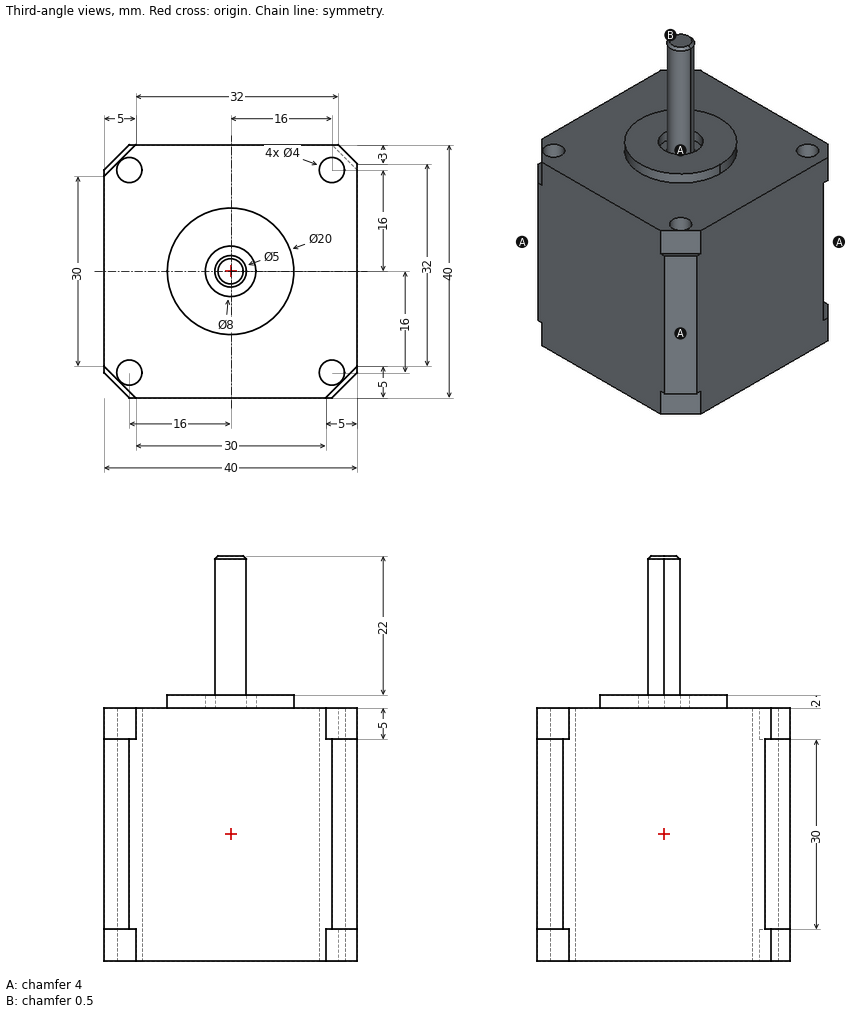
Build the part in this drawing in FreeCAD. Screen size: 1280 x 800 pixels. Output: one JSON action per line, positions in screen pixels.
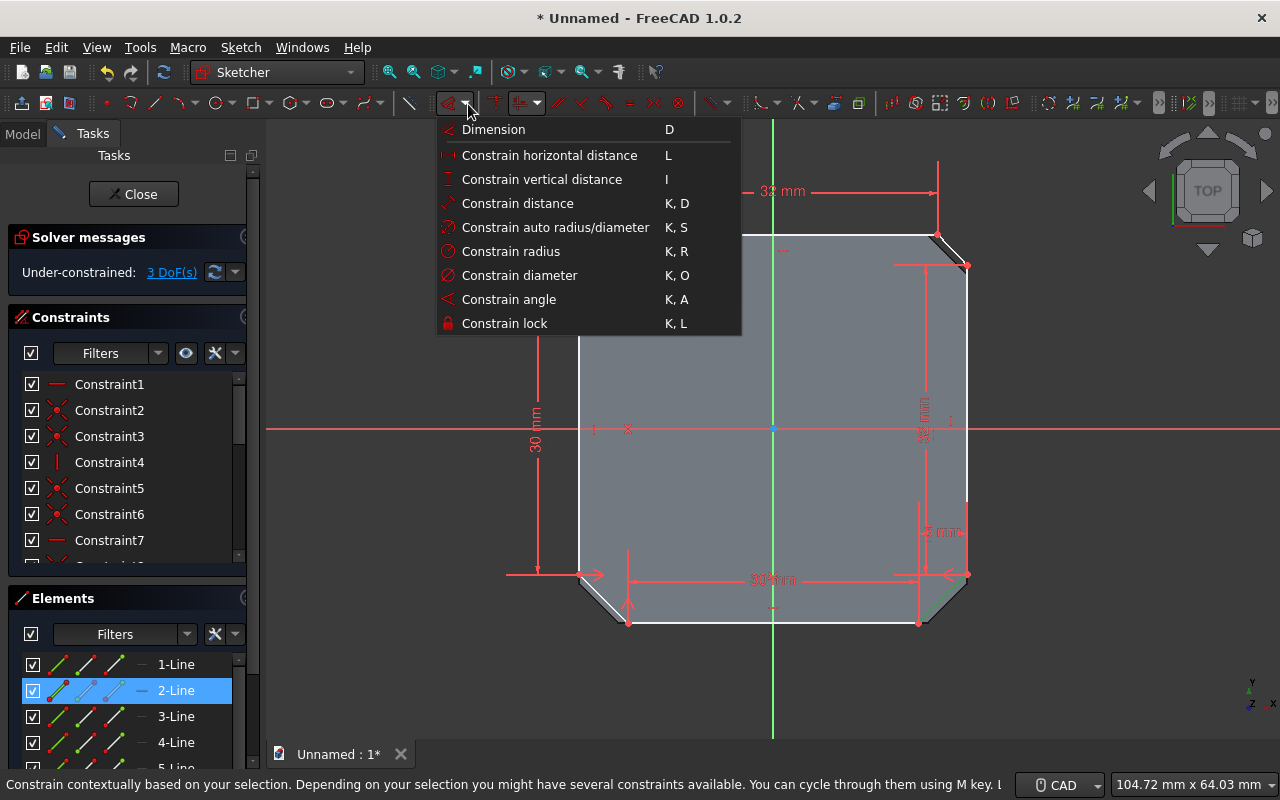
{"action": "left_click", "coordinate": [589, 179]}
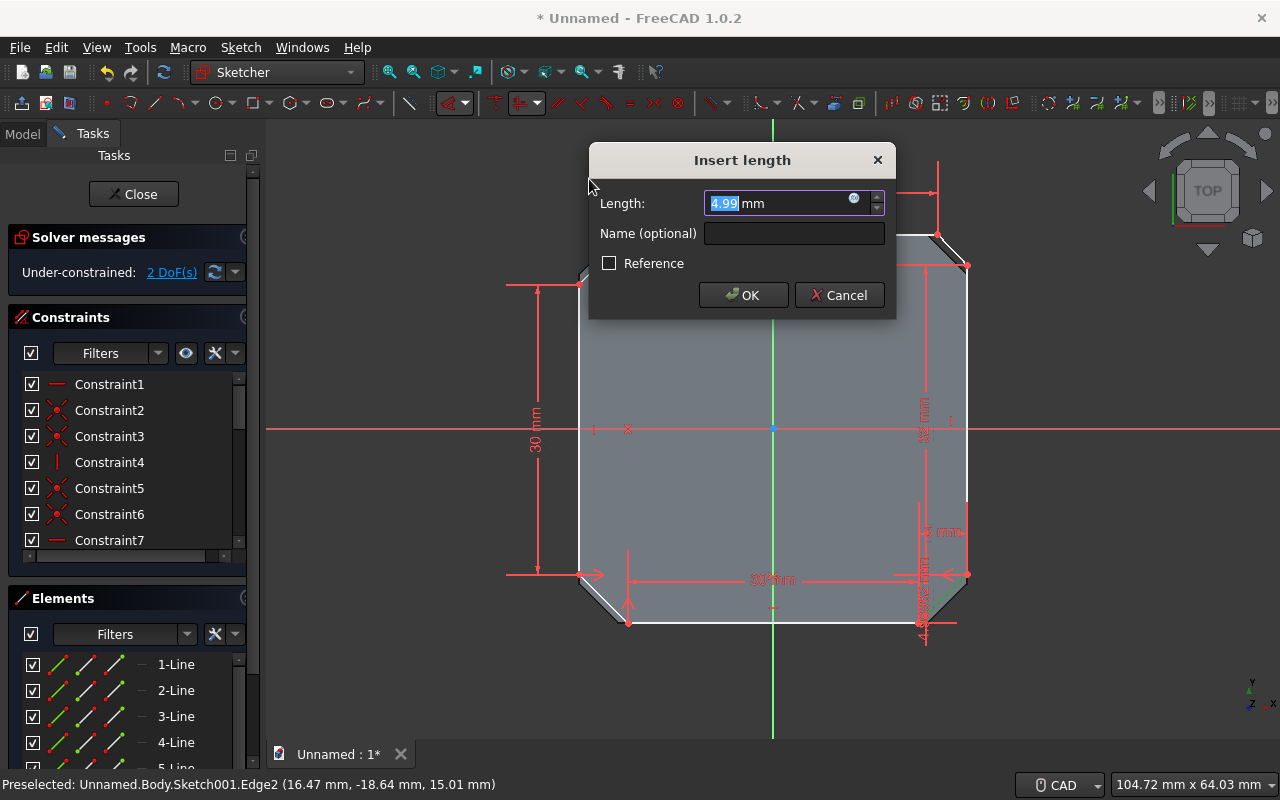
{"action": "type", "text": "5"}
{"action": "key", "text": "Return"}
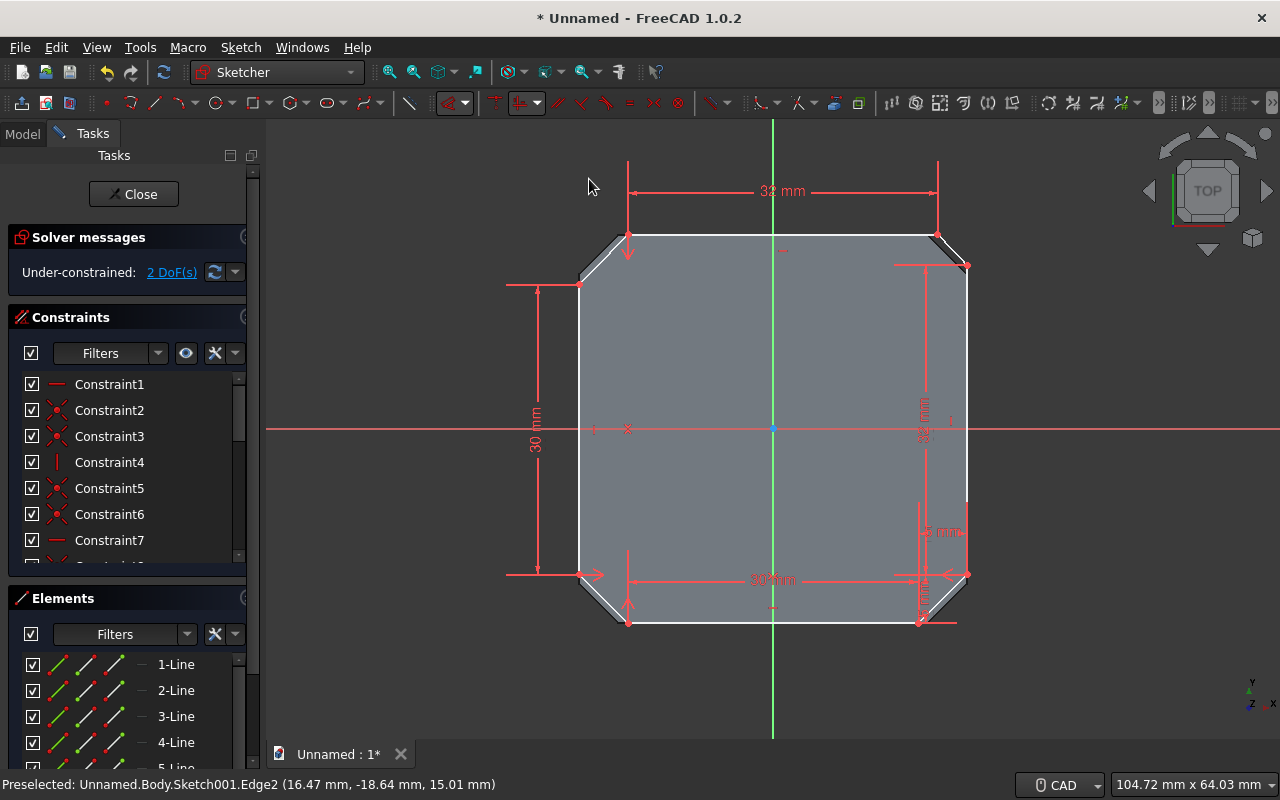
{"action": "scroll", "coordinate": [958, 256], "scroll_direction": "up", "scroll_amount": 2}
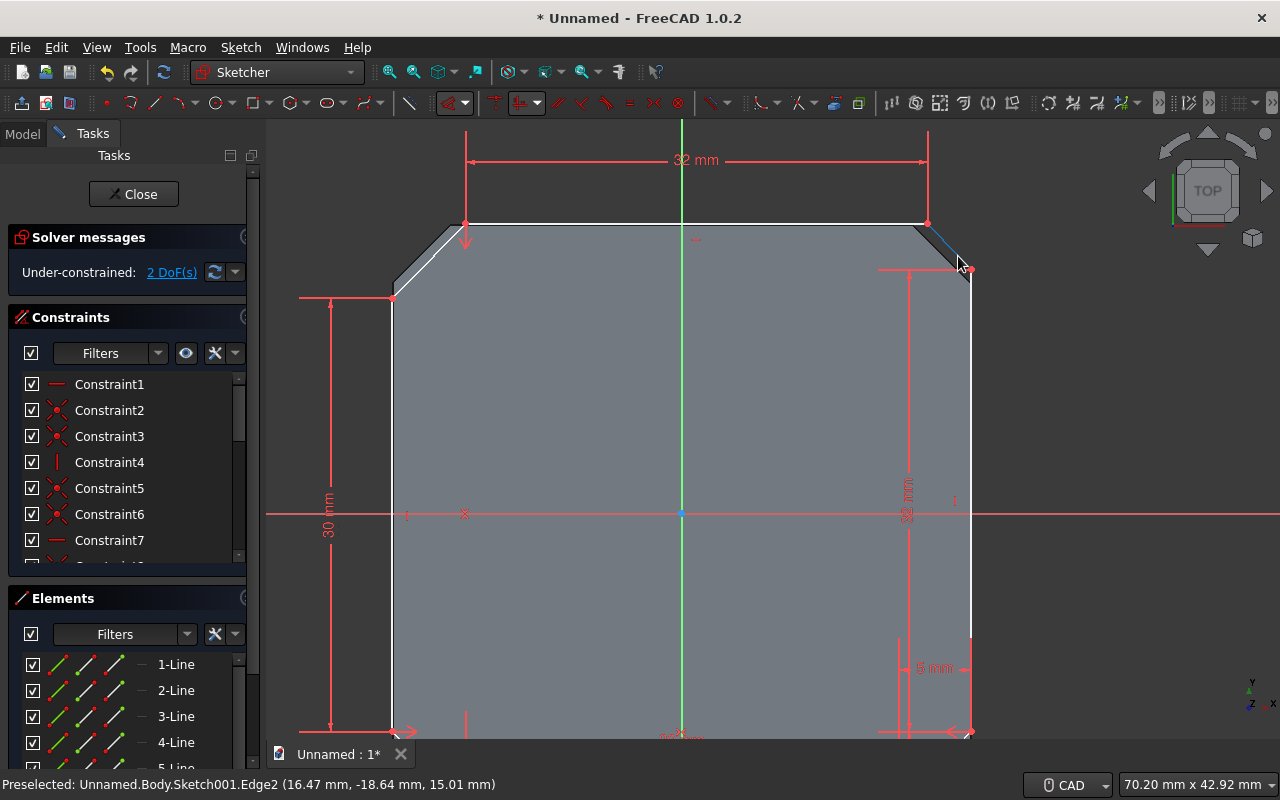
{"action": "left_click", "coordinate": [958, 256]}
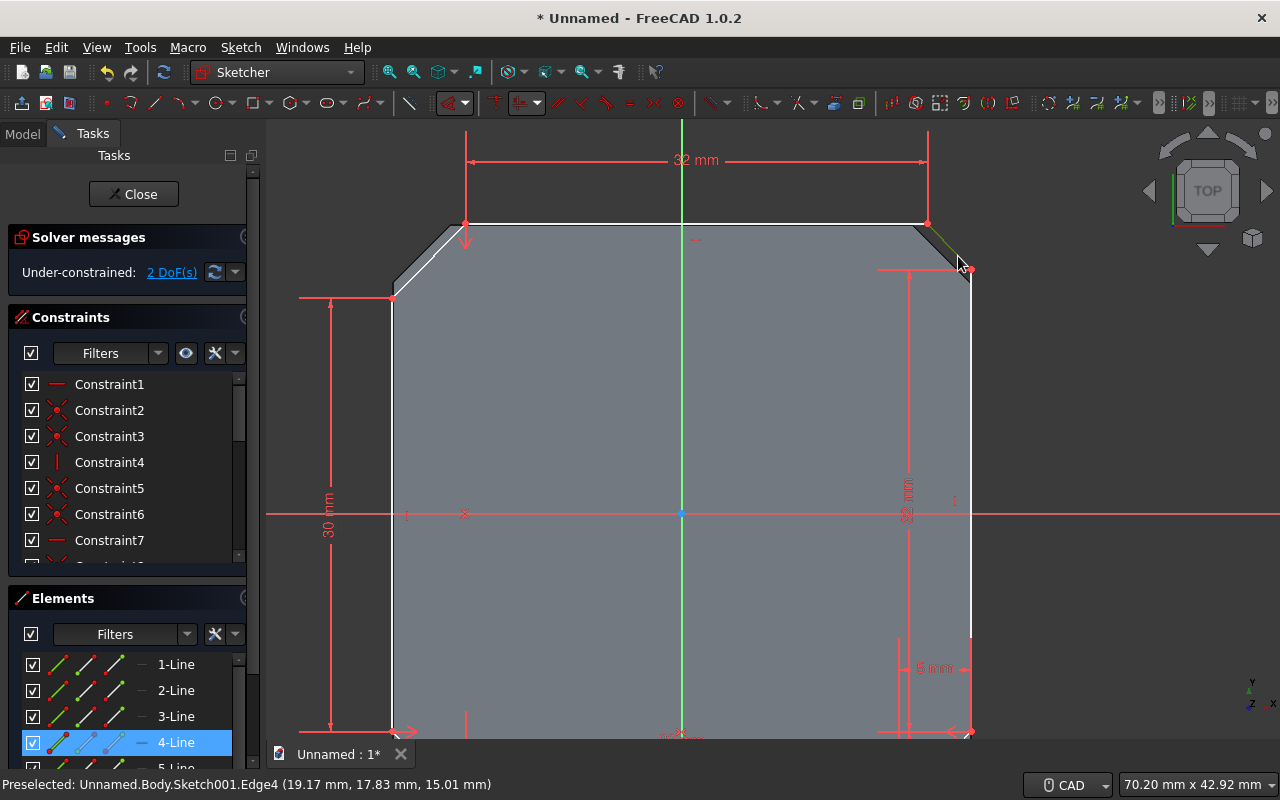
{"action": "key", "text": "i"}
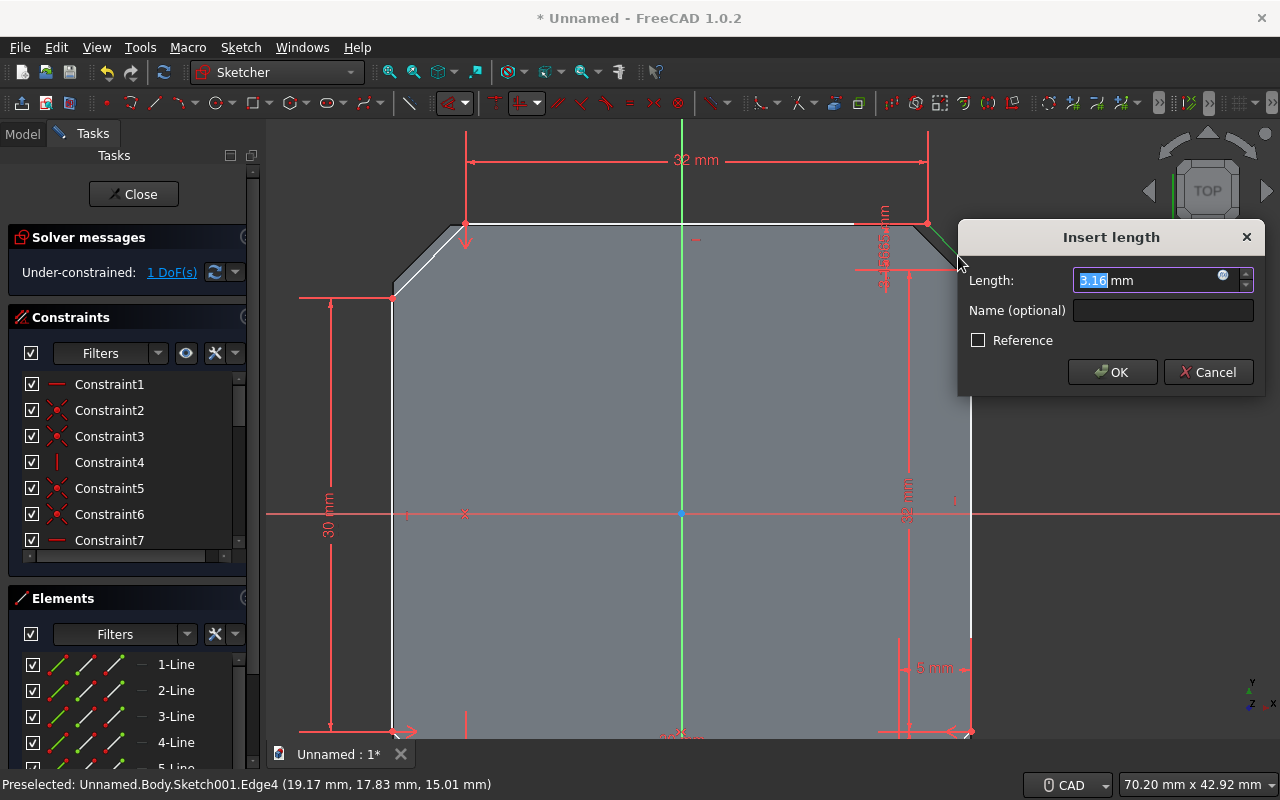
{"action": "type", "text": "3"}
{"action": "key", "text": "Return"}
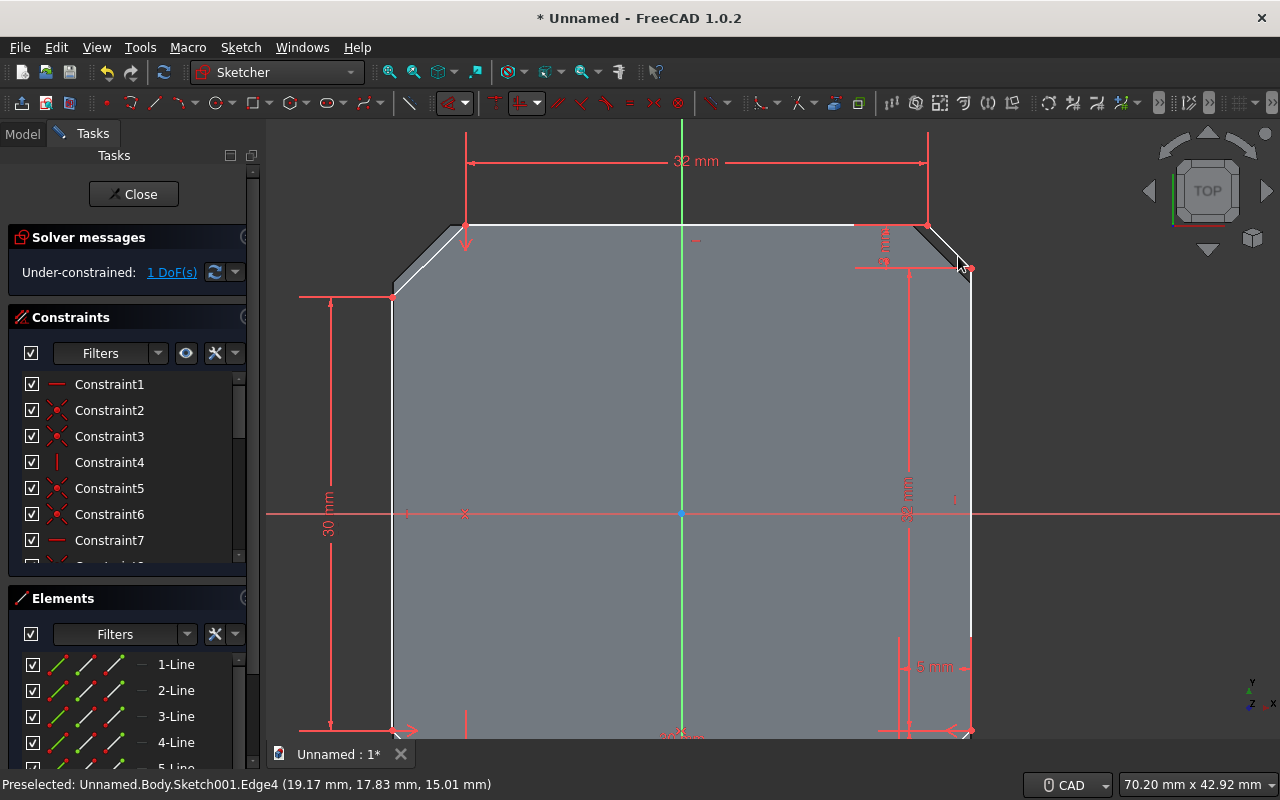
{"action": "left_click", "coordinate": [444, 247]}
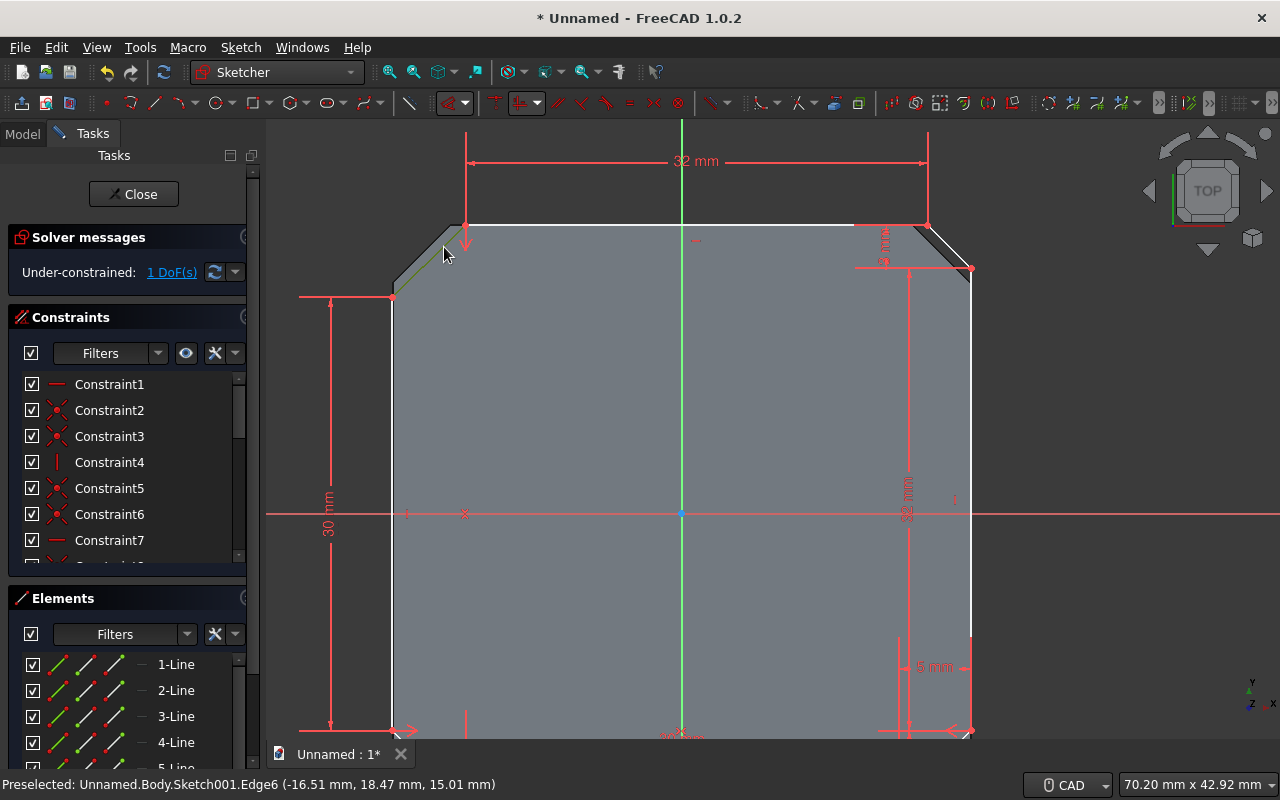
{"action": "key", "text": "l"}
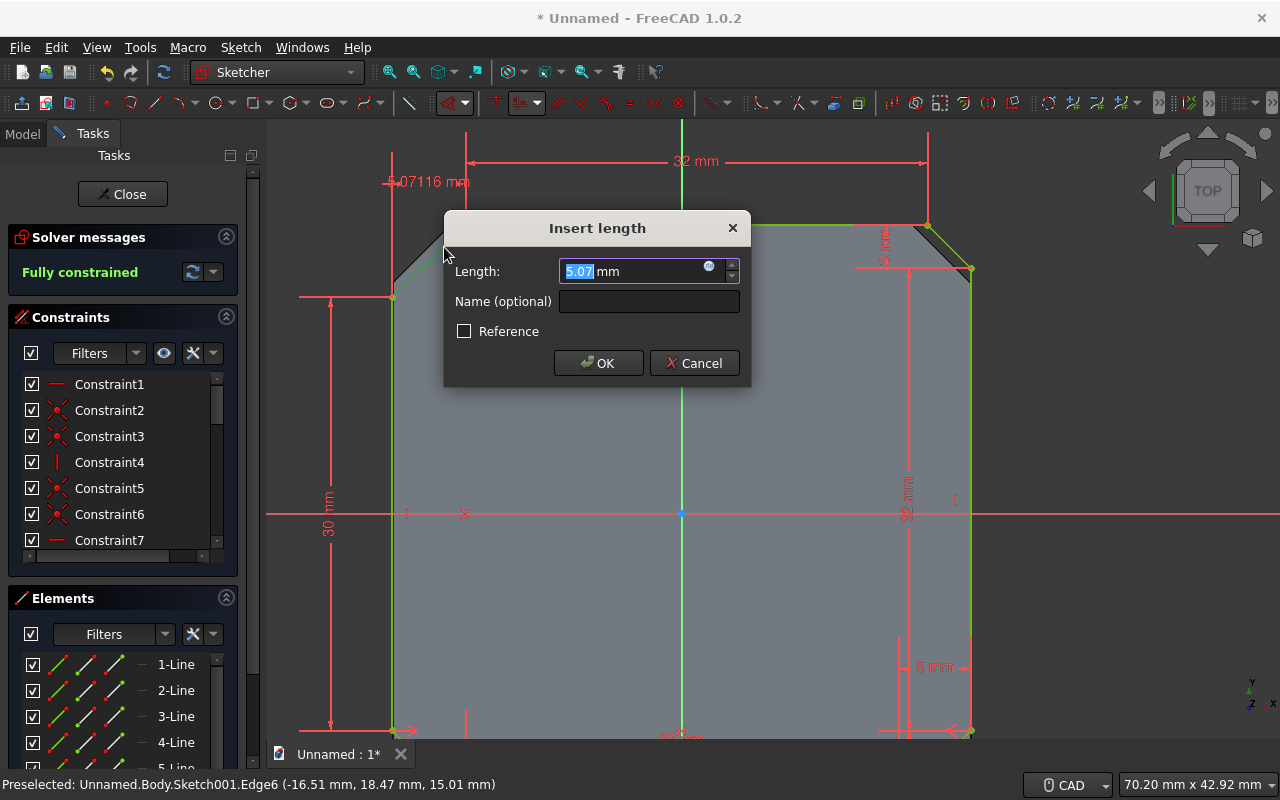
{"action": "type", "text": "5"}
{"action": "key", "text": "Return"}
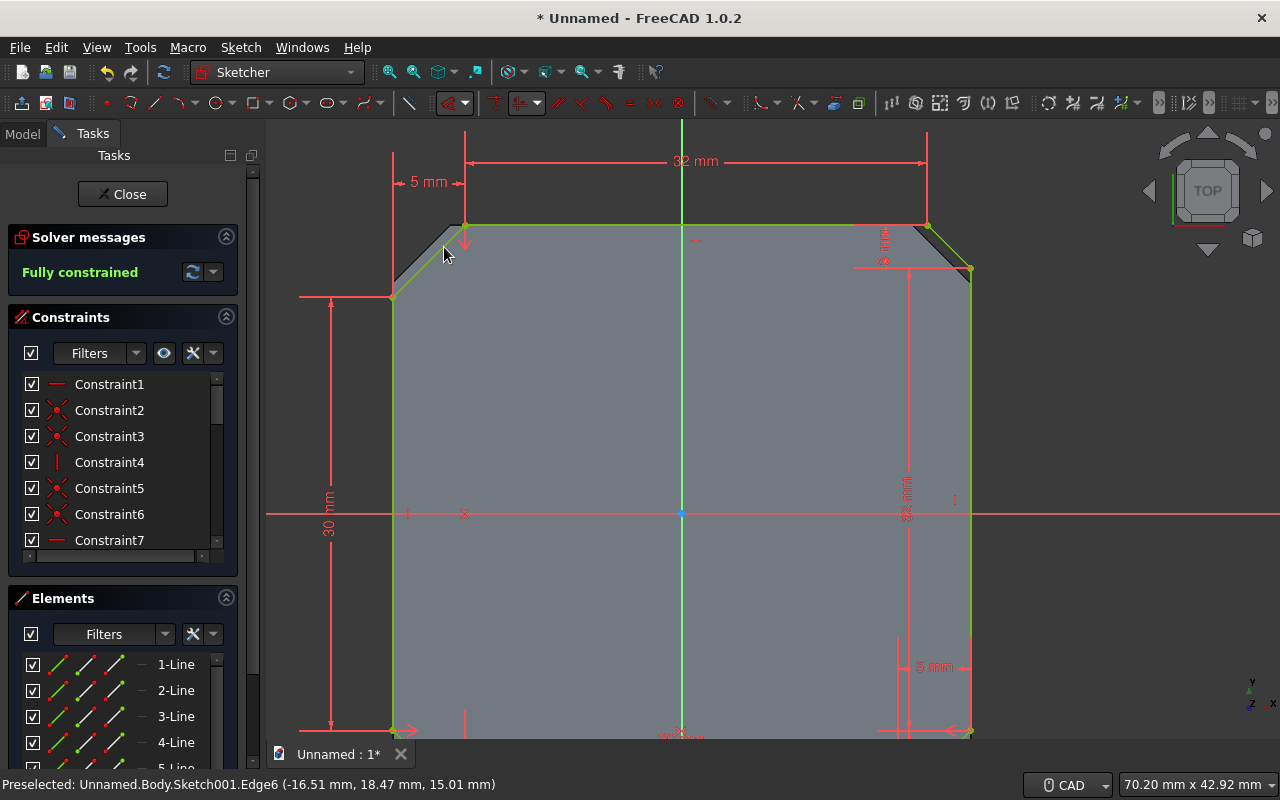
{"action": "left_click", "coordinate": [123, 194]}